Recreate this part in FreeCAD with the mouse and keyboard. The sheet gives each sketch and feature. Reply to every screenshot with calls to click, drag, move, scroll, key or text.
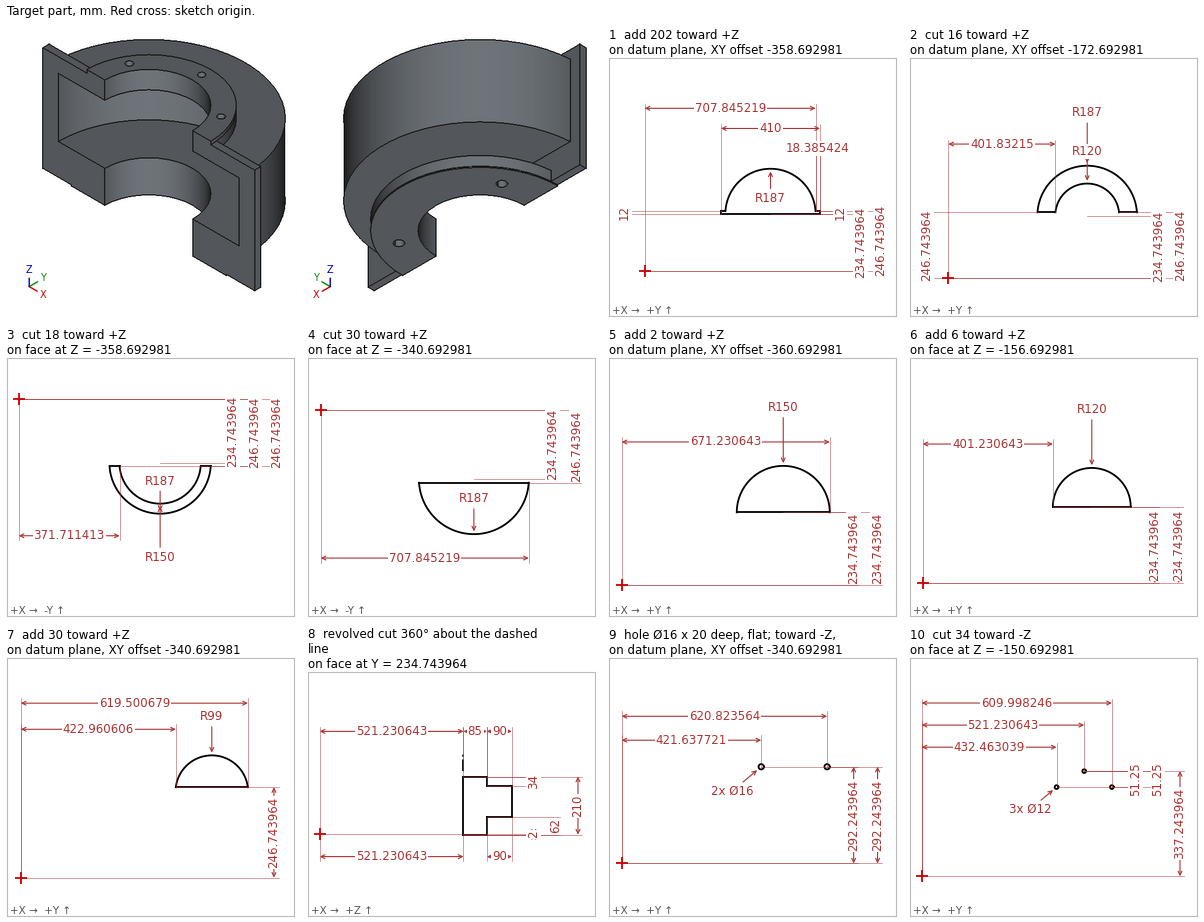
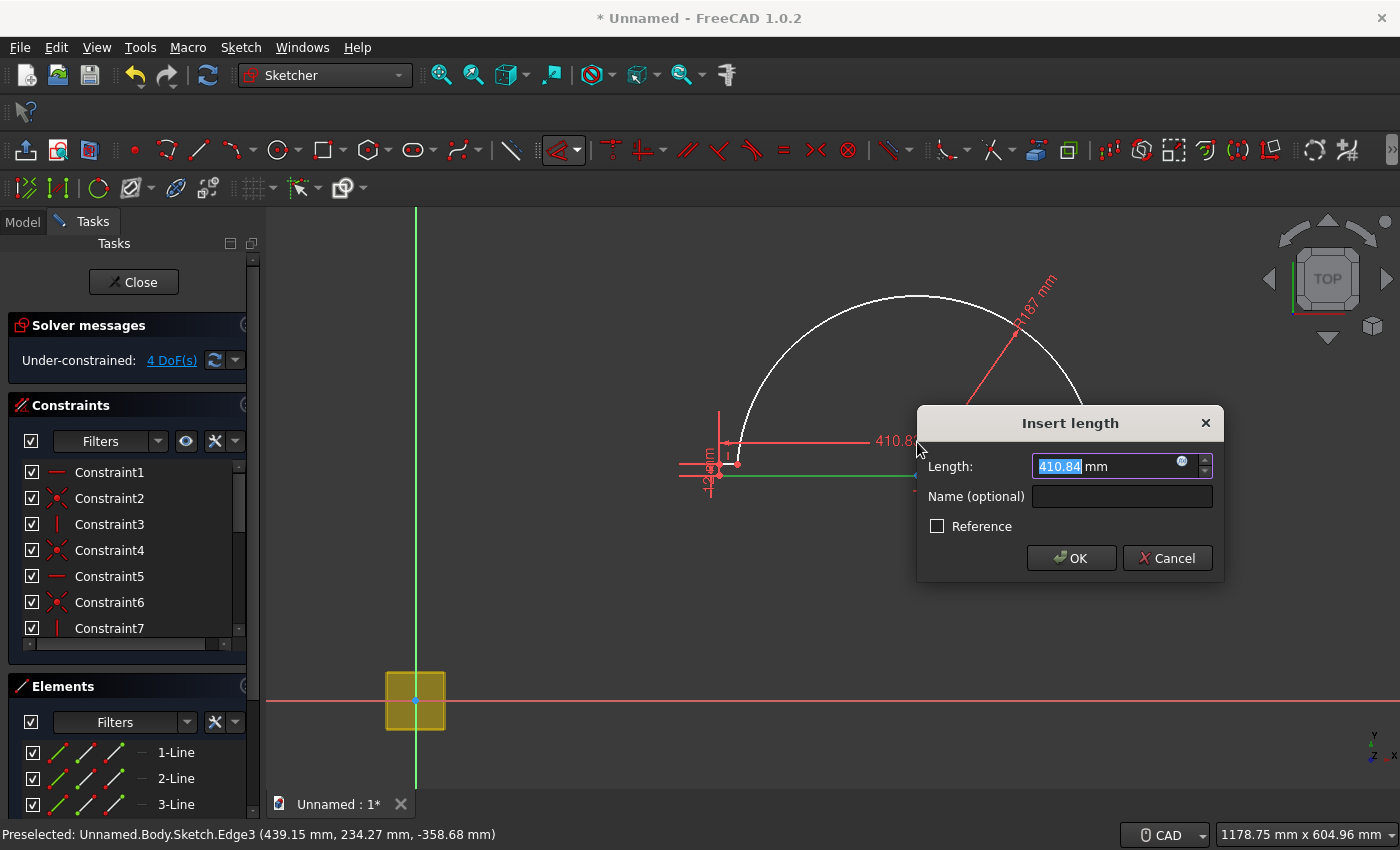
text(410)
key(Return)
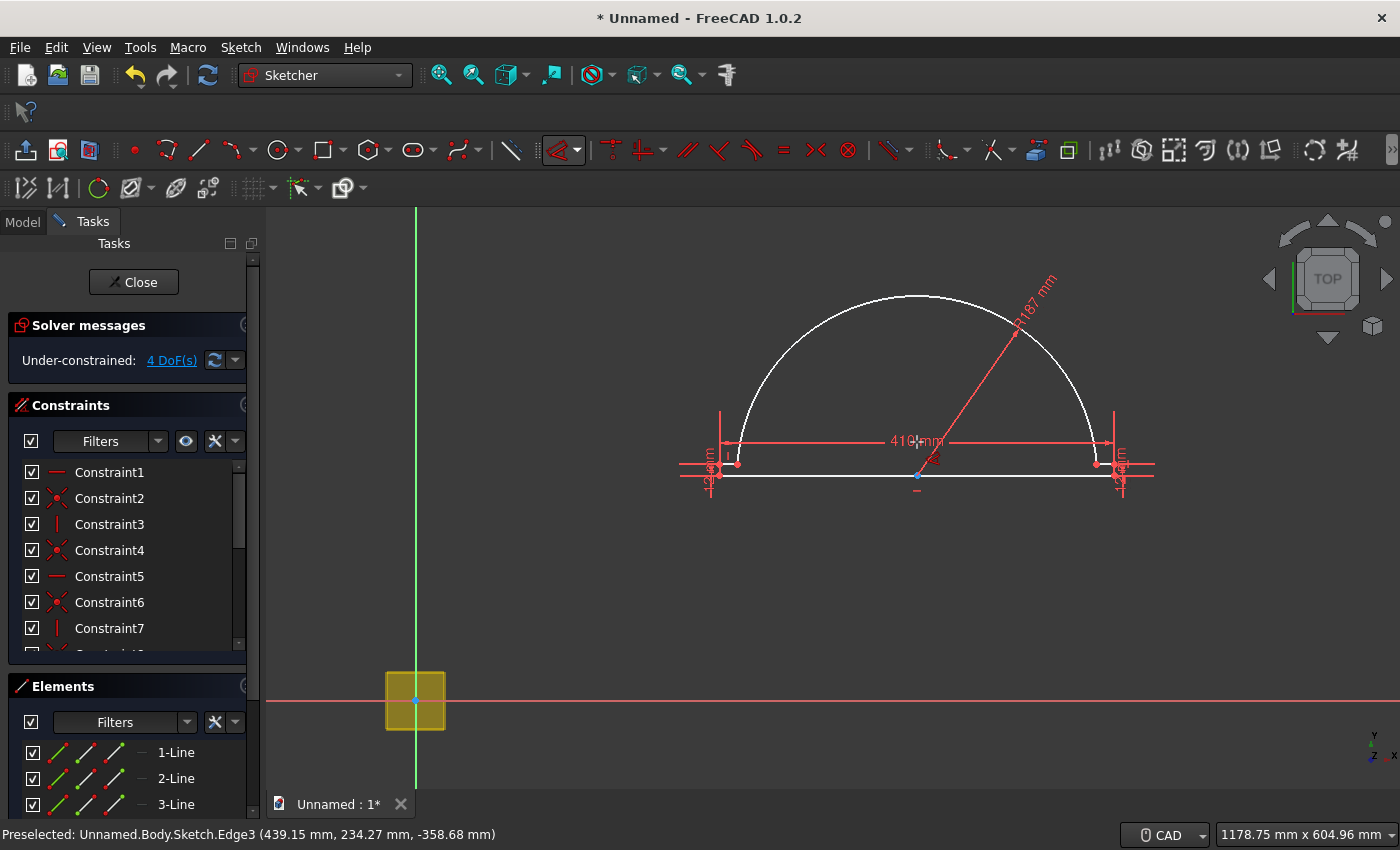
scroll(1105, 464, up, 5)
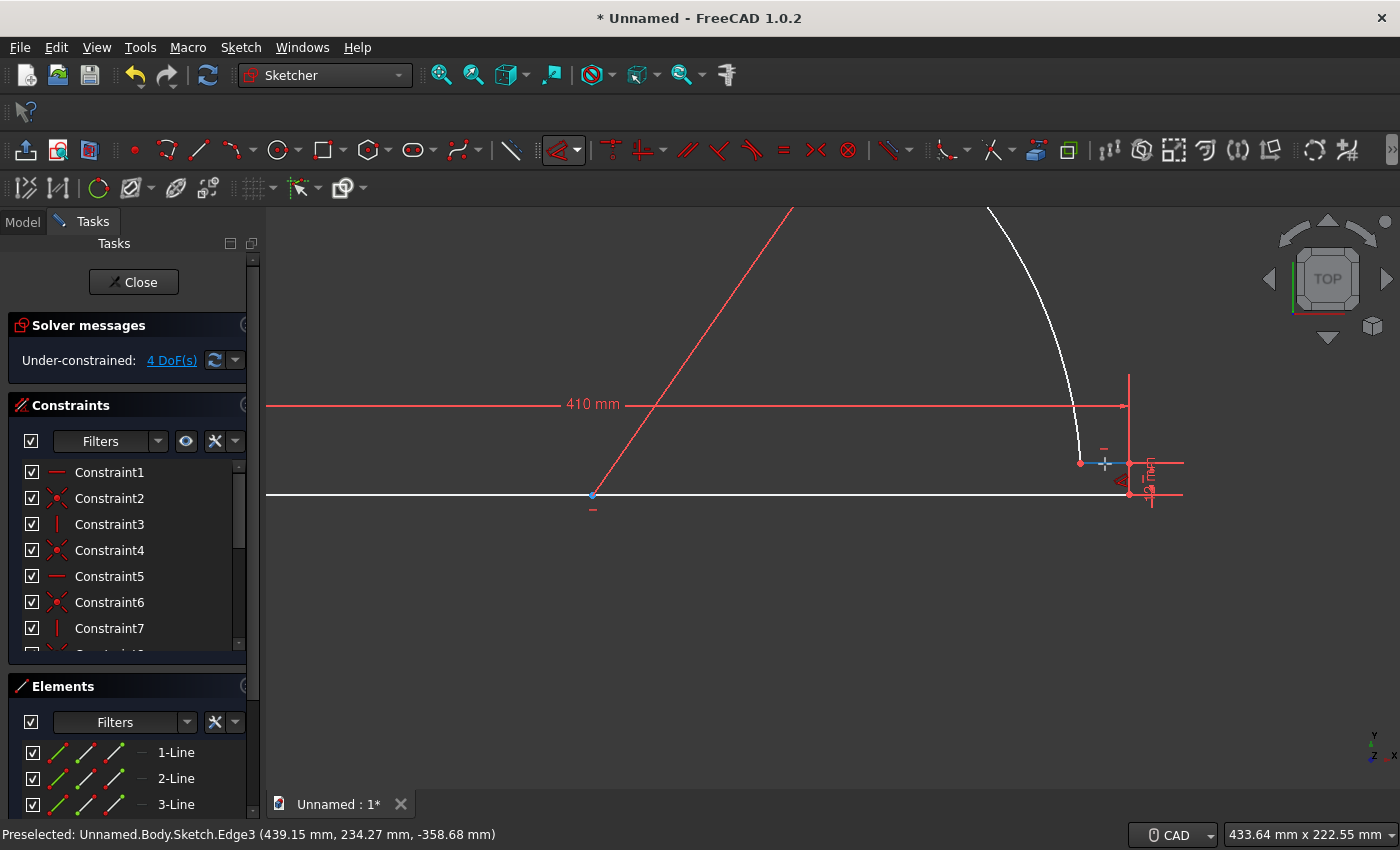
click(1105, 463)
click(1105, 429)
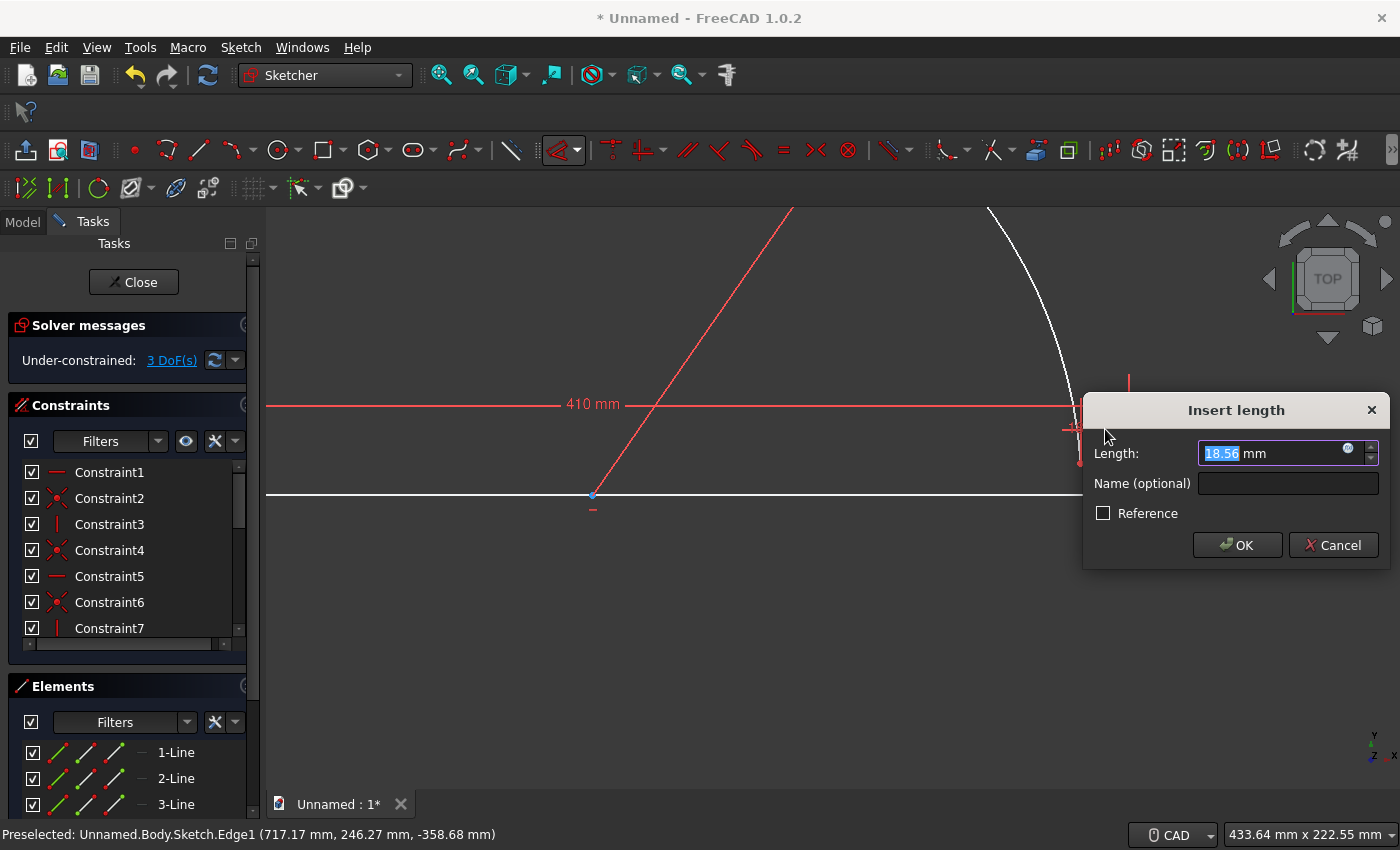
text(18.385424)
key(Return)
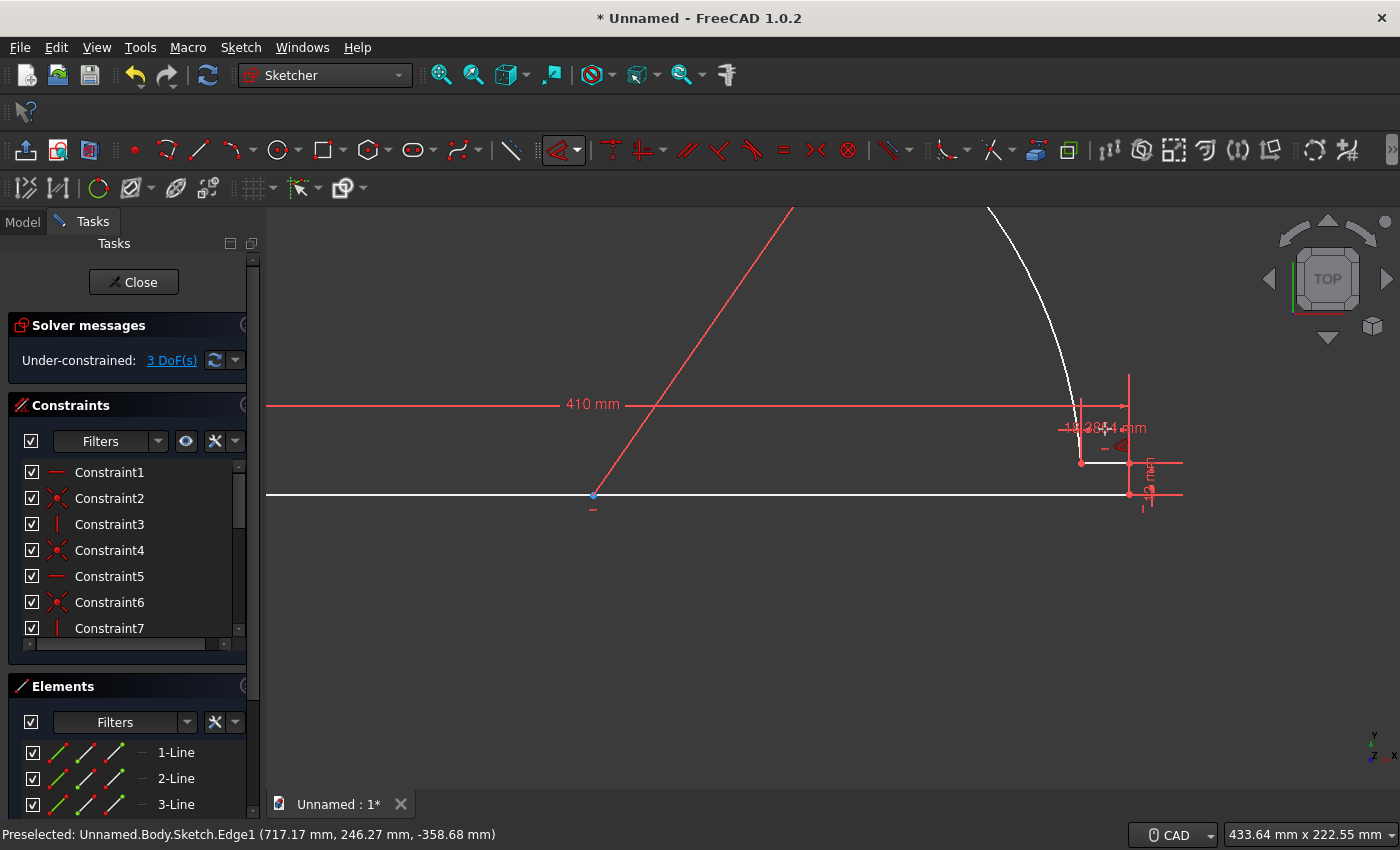
click(1081, 463)
click(688, 429)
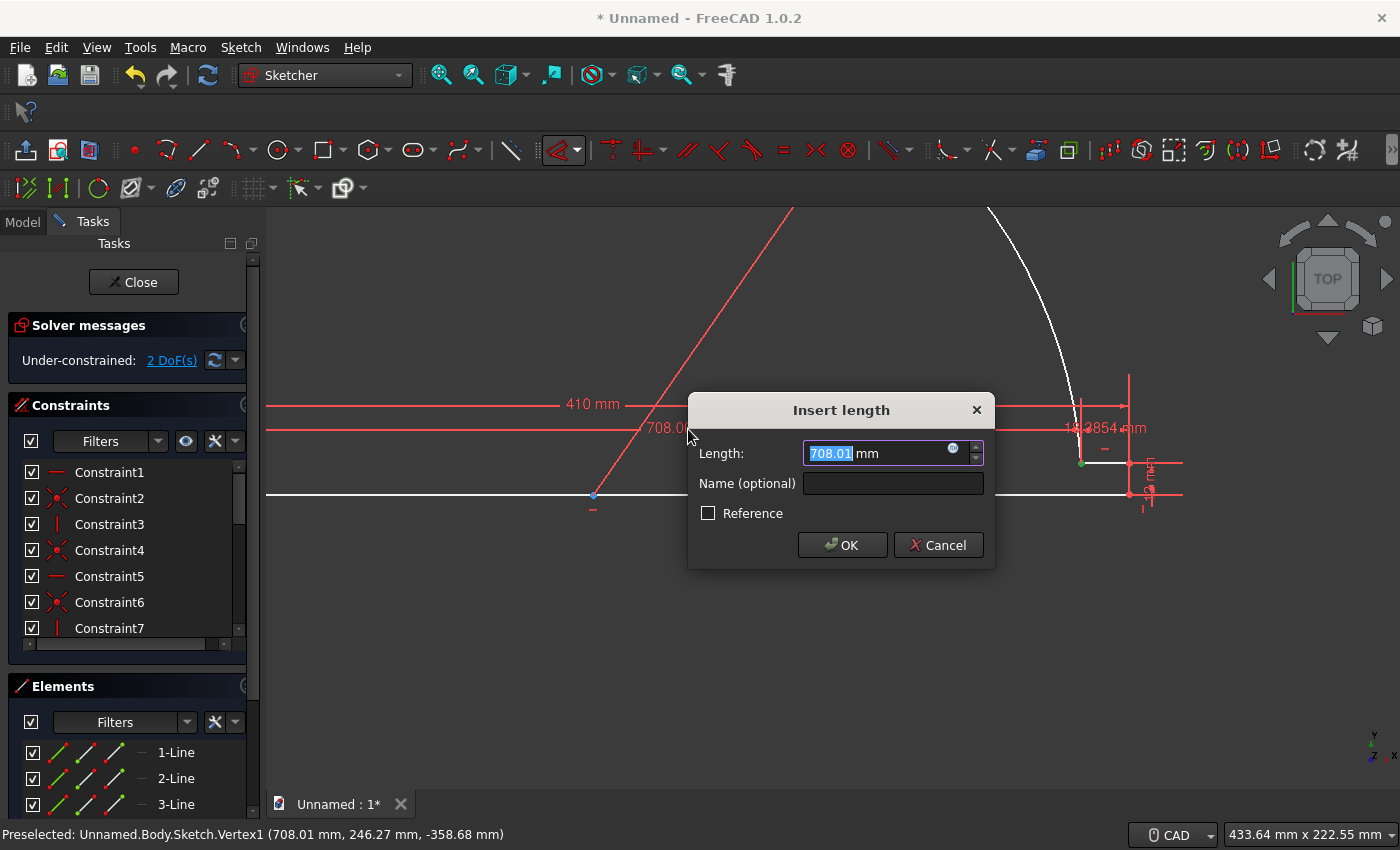
text(707.845219)
key(Return)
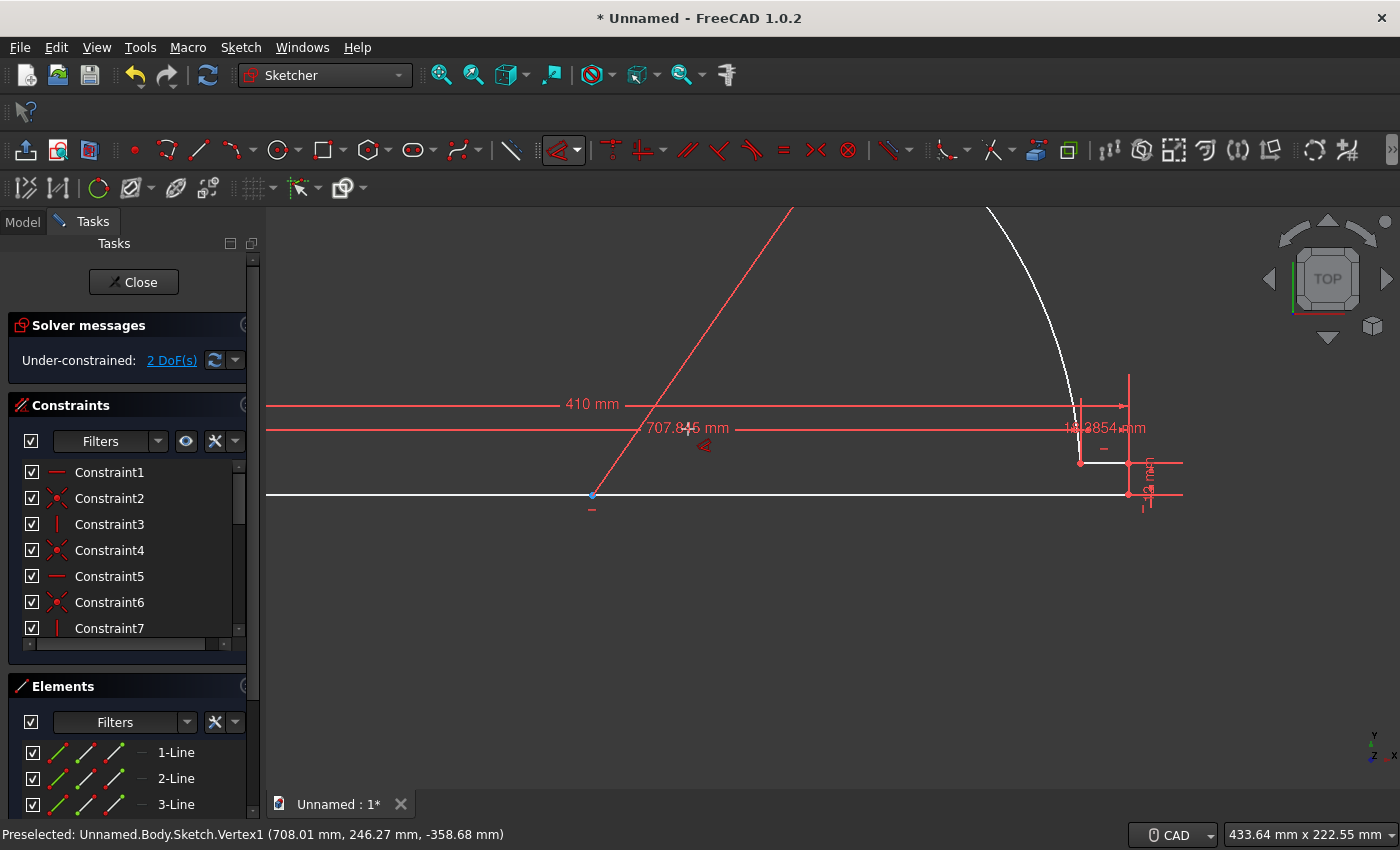
click(1081, 463)
click(1115, 612)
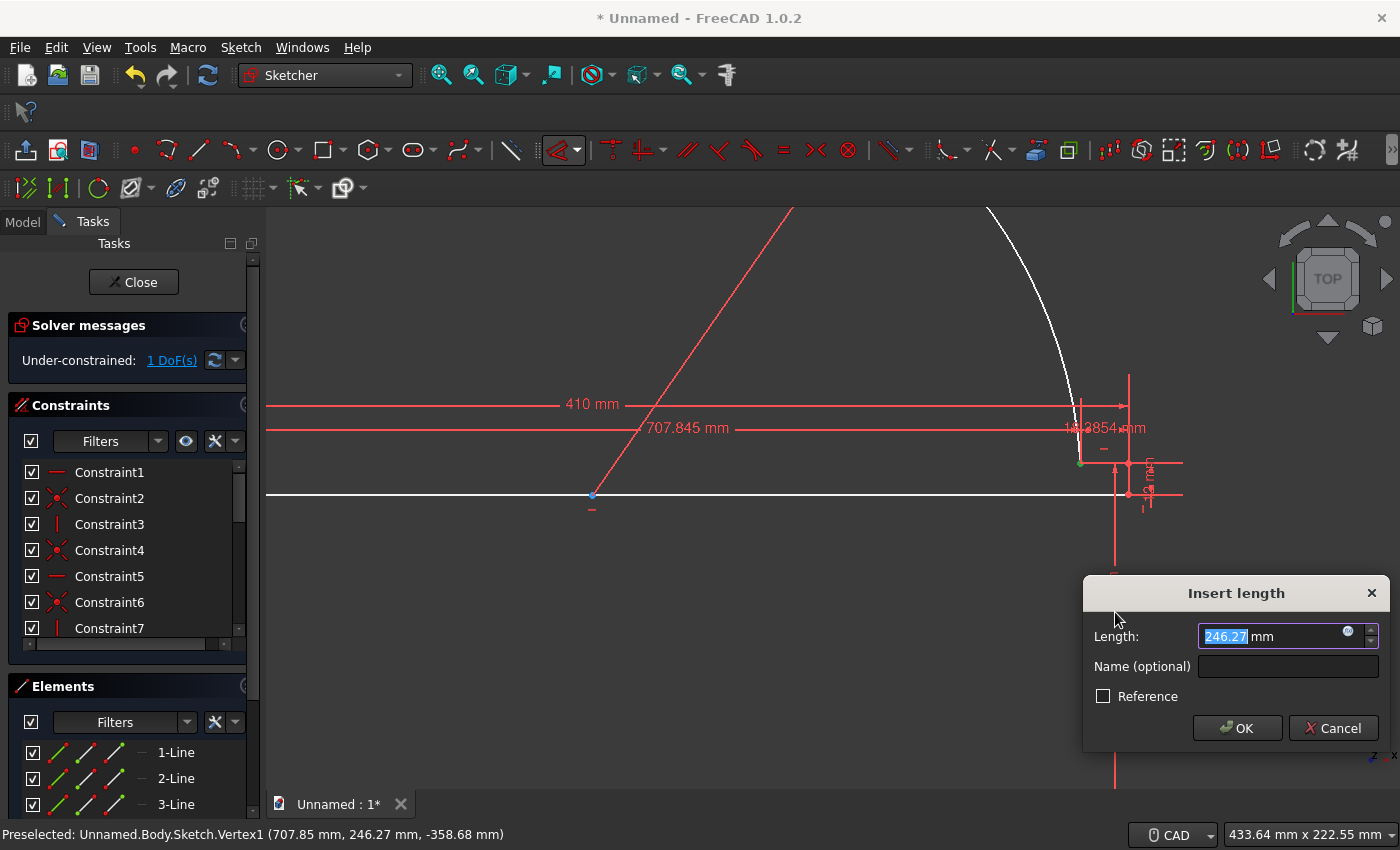
text(246.743964)
key(Return)